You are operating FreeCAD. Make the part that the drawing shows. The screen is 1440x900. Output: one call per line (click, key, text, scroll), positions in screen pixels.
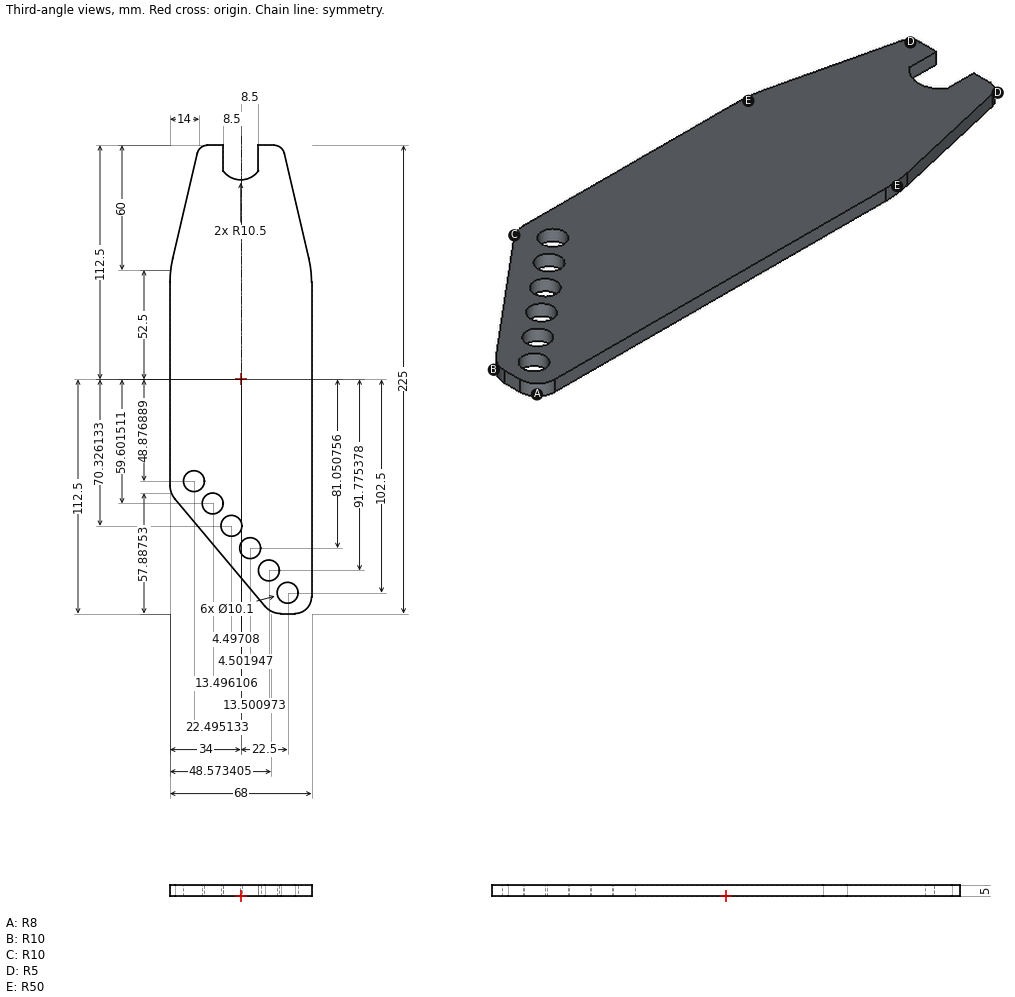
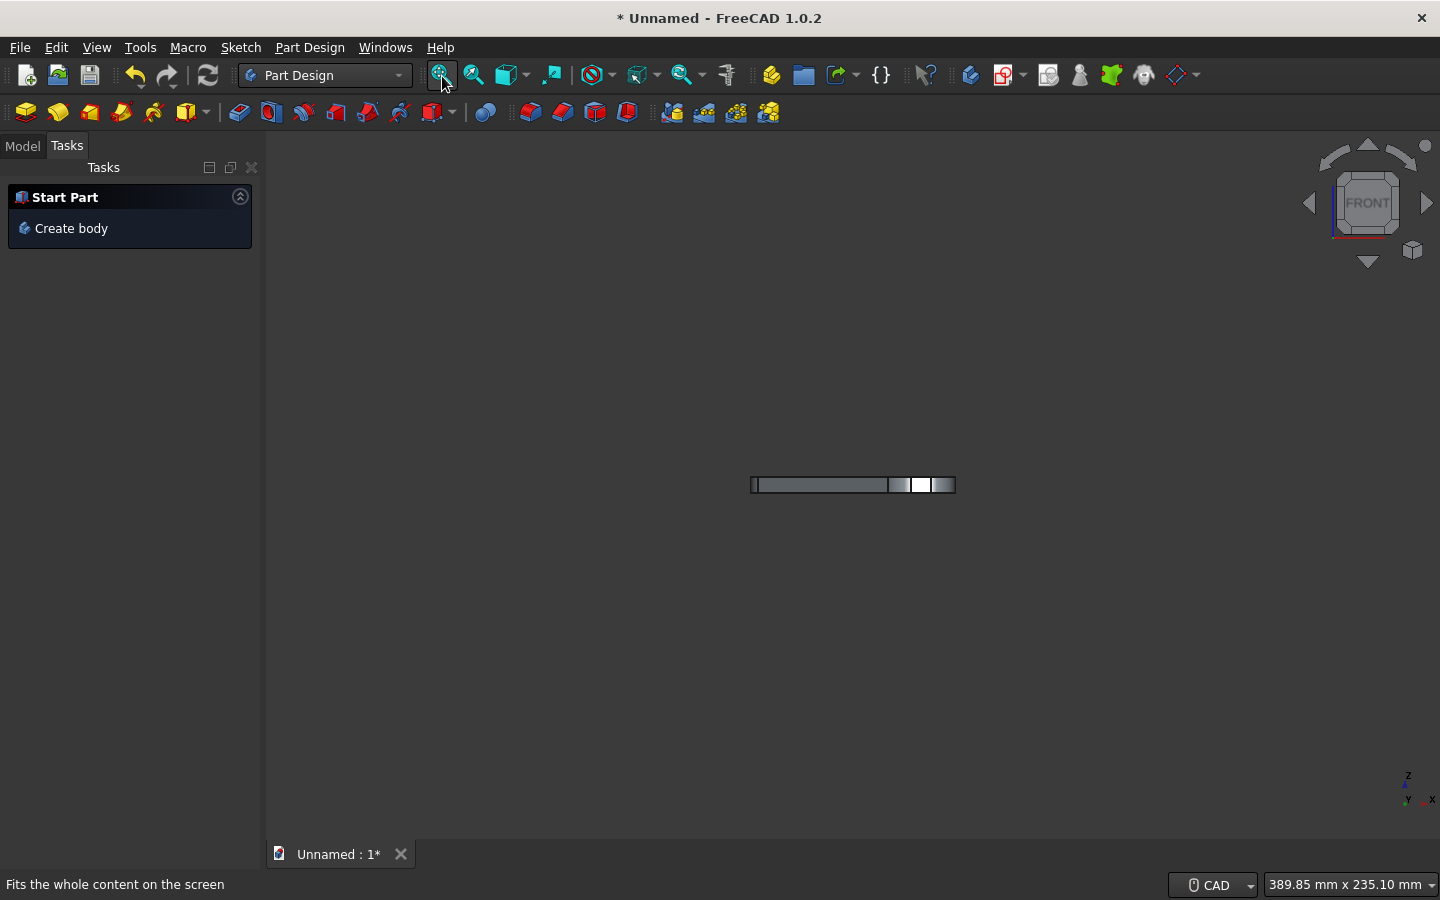
key(3)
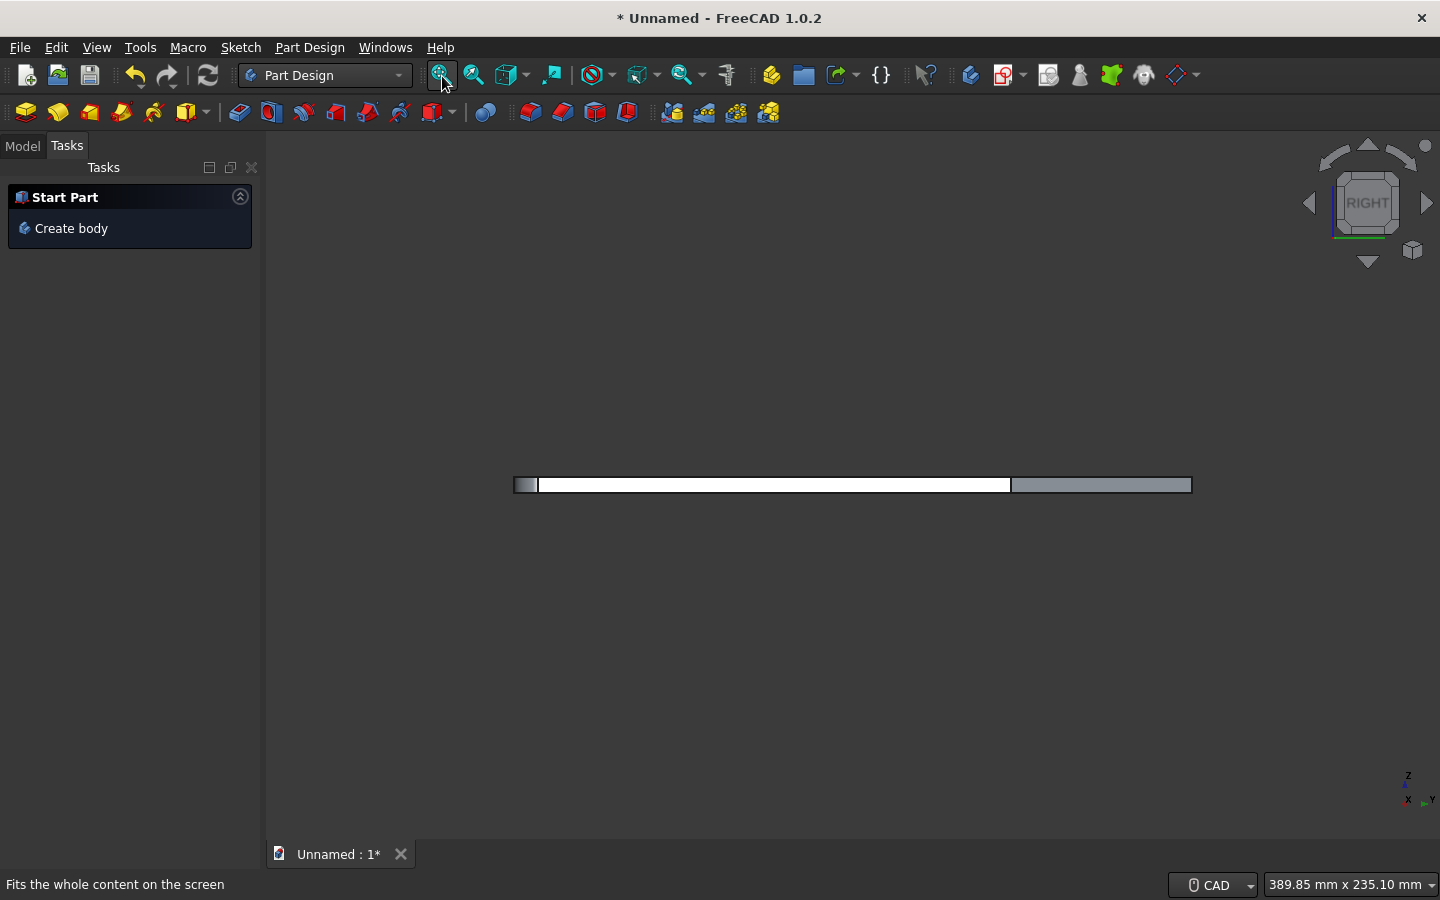
scroll(1192, 484, up, 5)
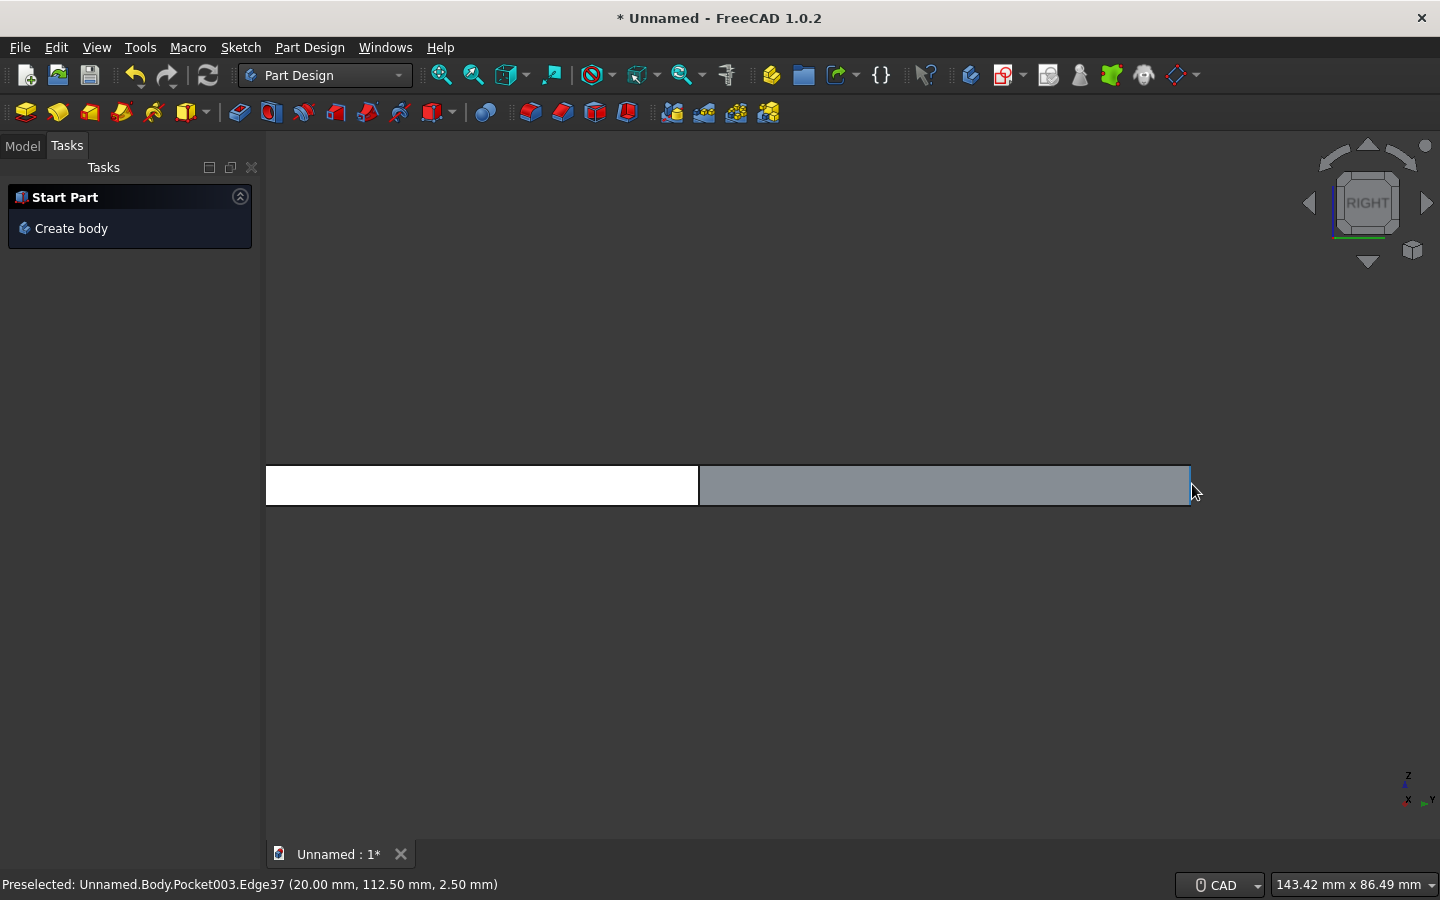
key(v)
key(f)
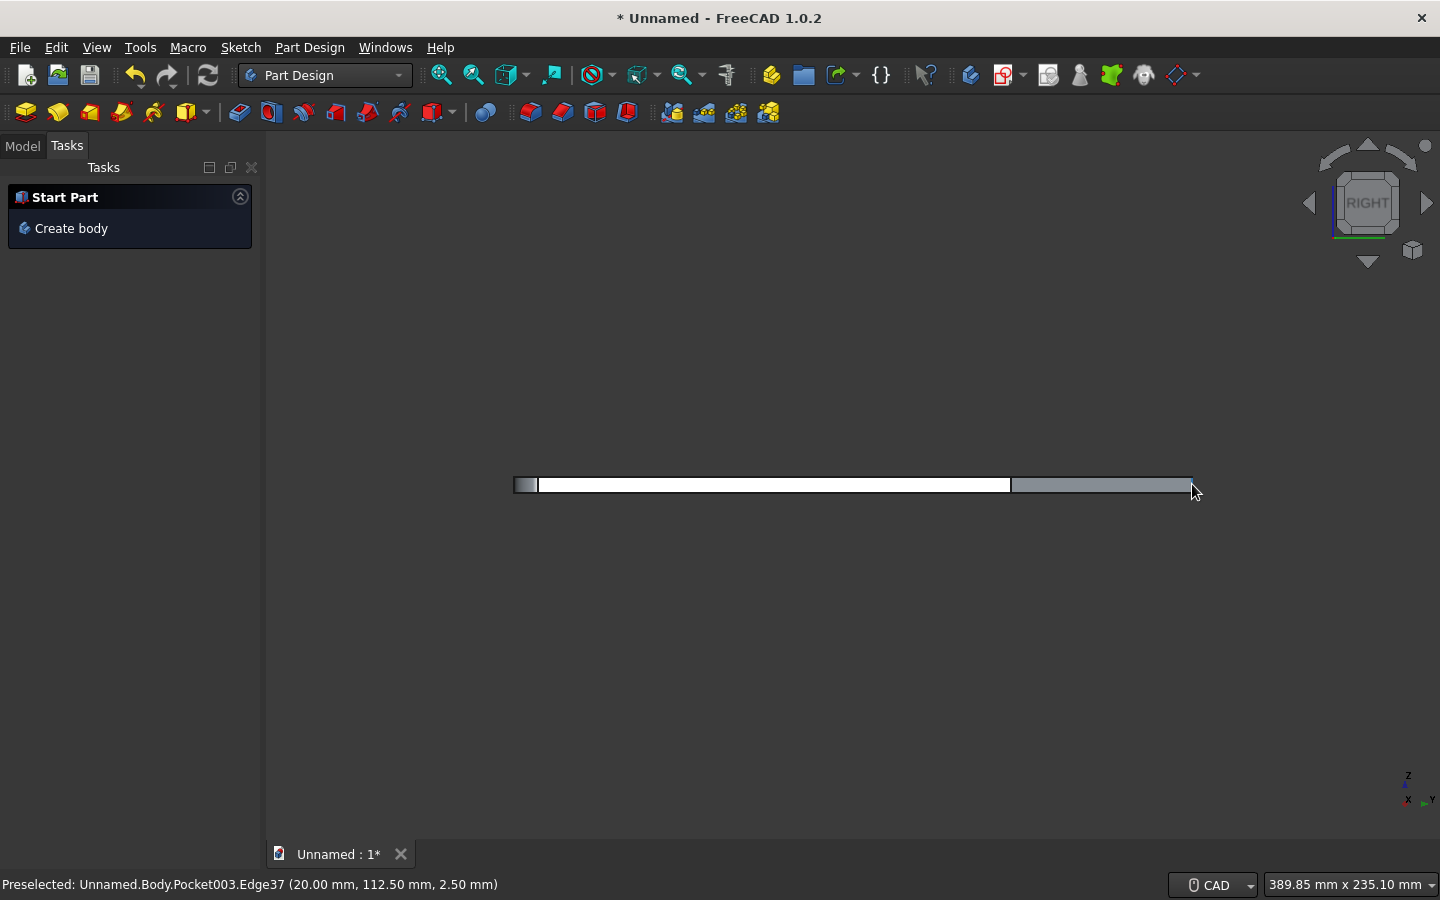
key(5)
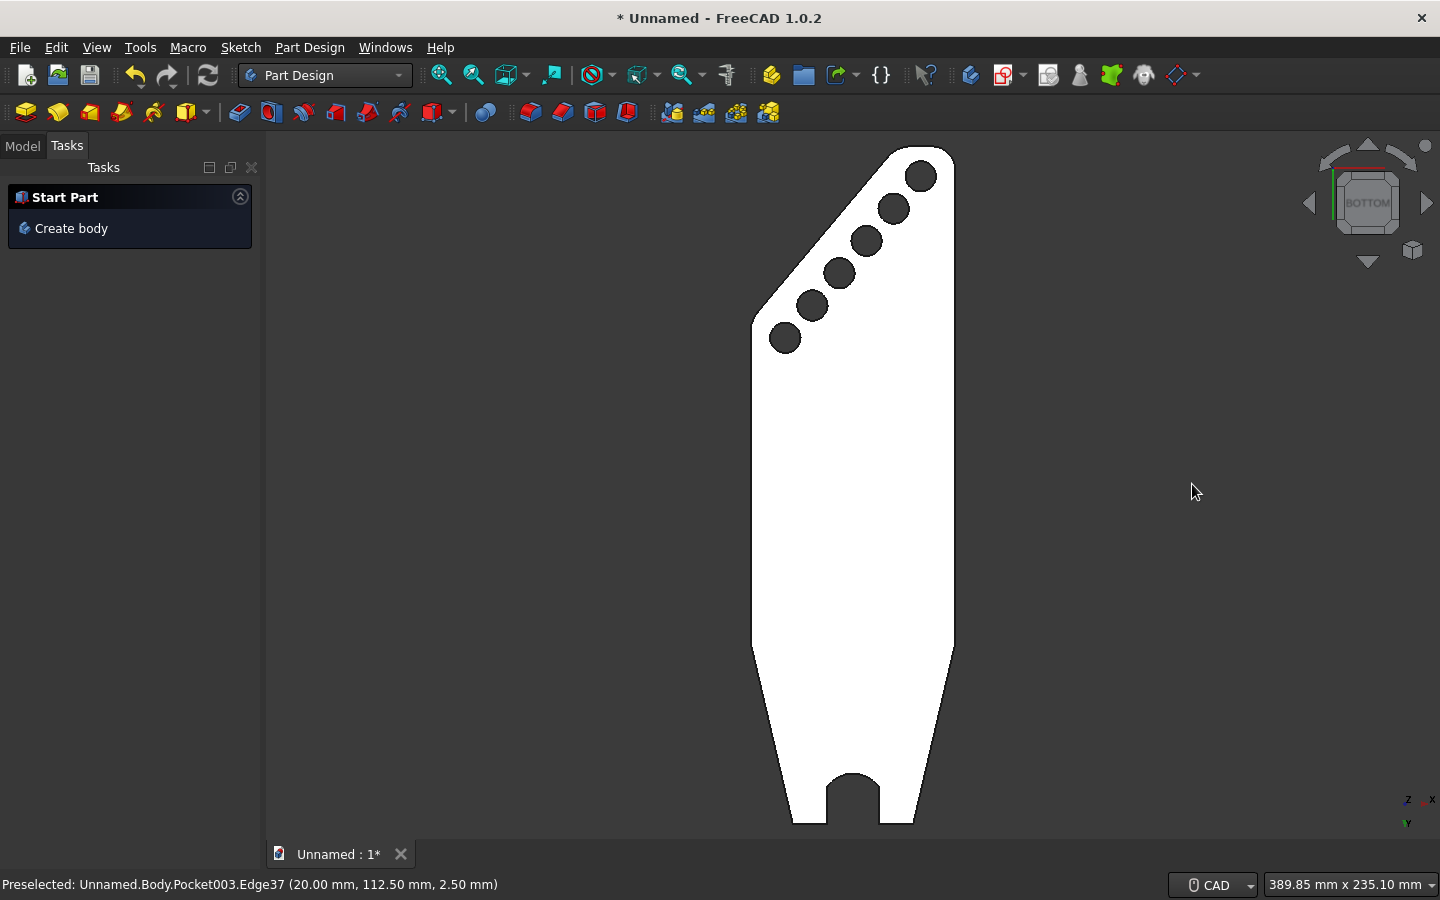
key(4)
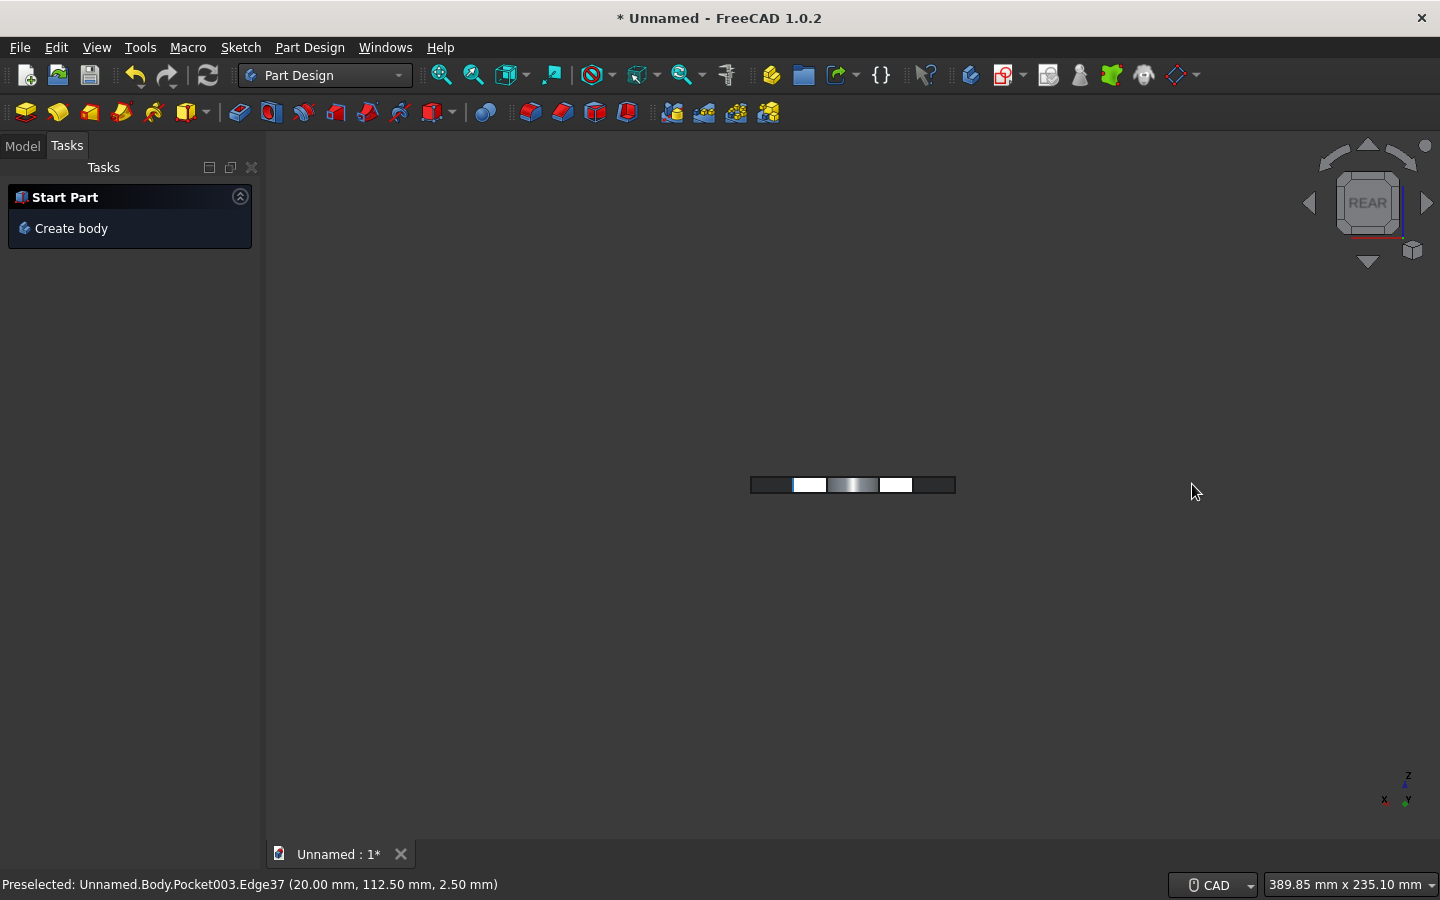
key(v)
key(f)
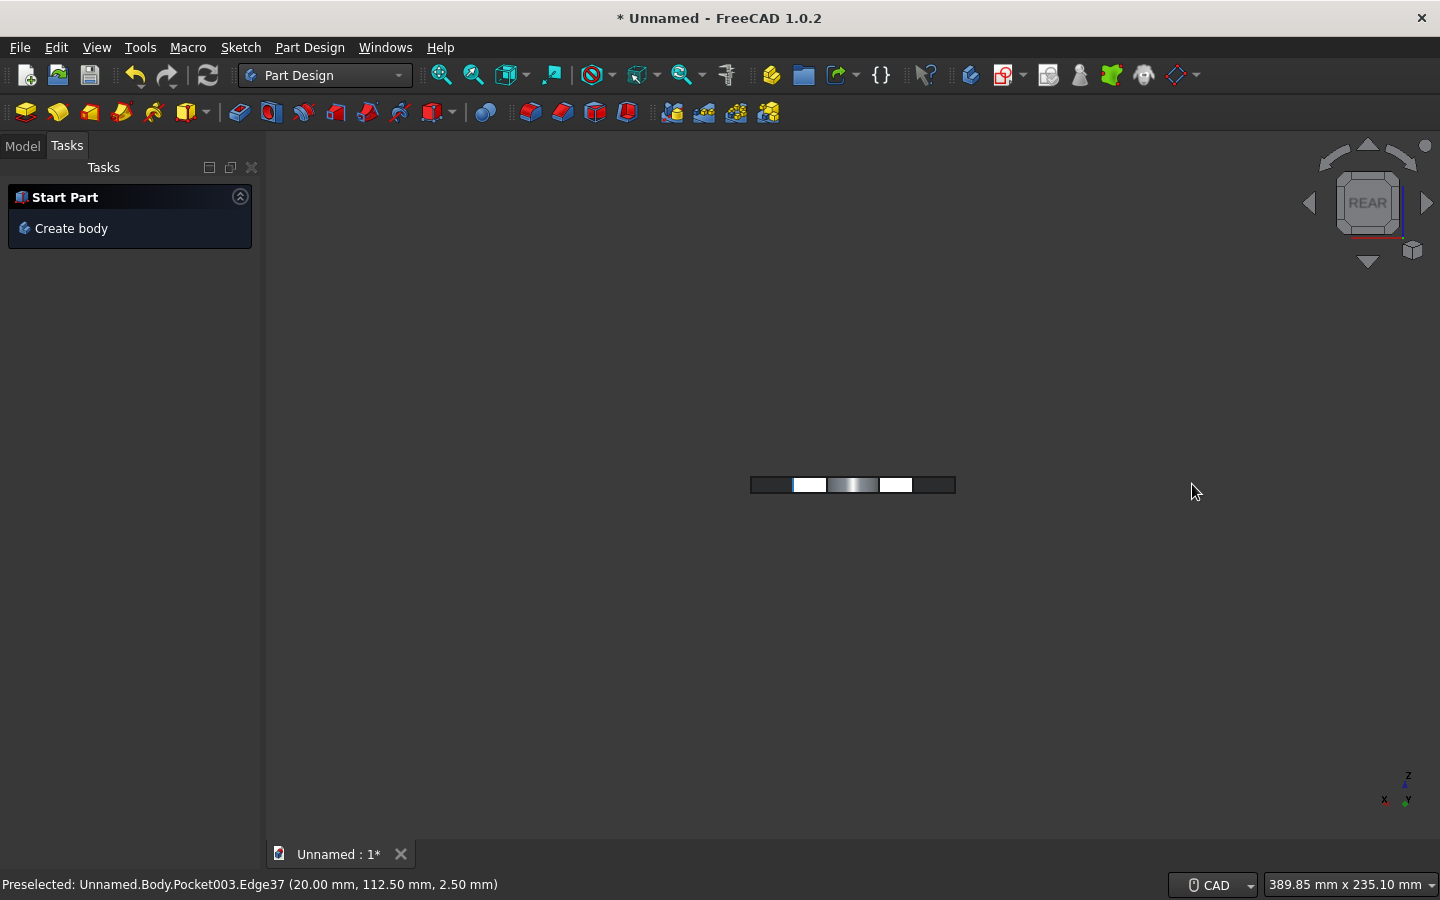
click(913, 484)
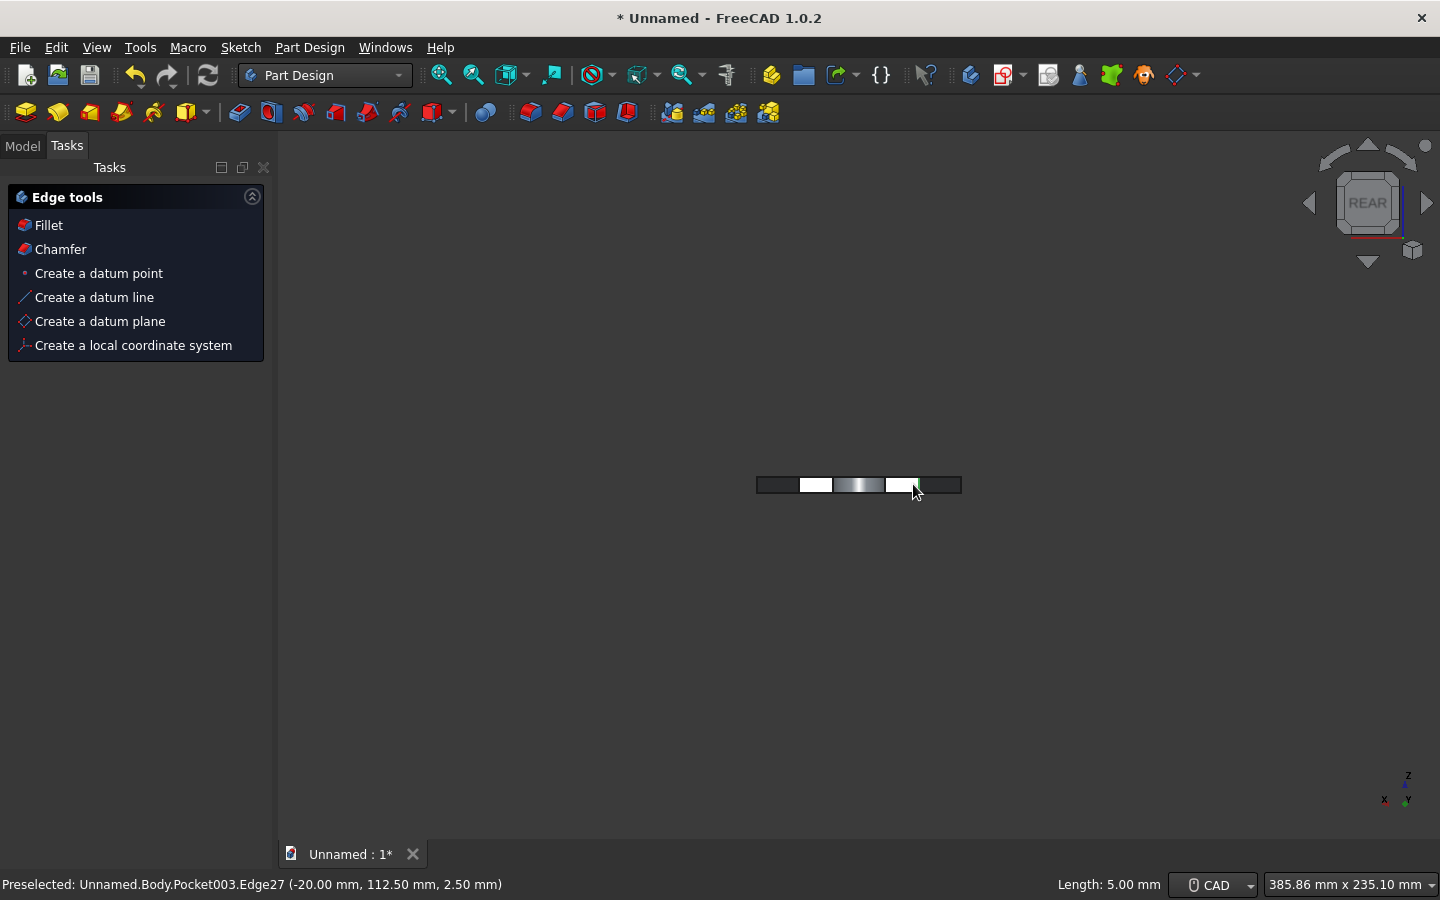
click(799, 484, ctrl)